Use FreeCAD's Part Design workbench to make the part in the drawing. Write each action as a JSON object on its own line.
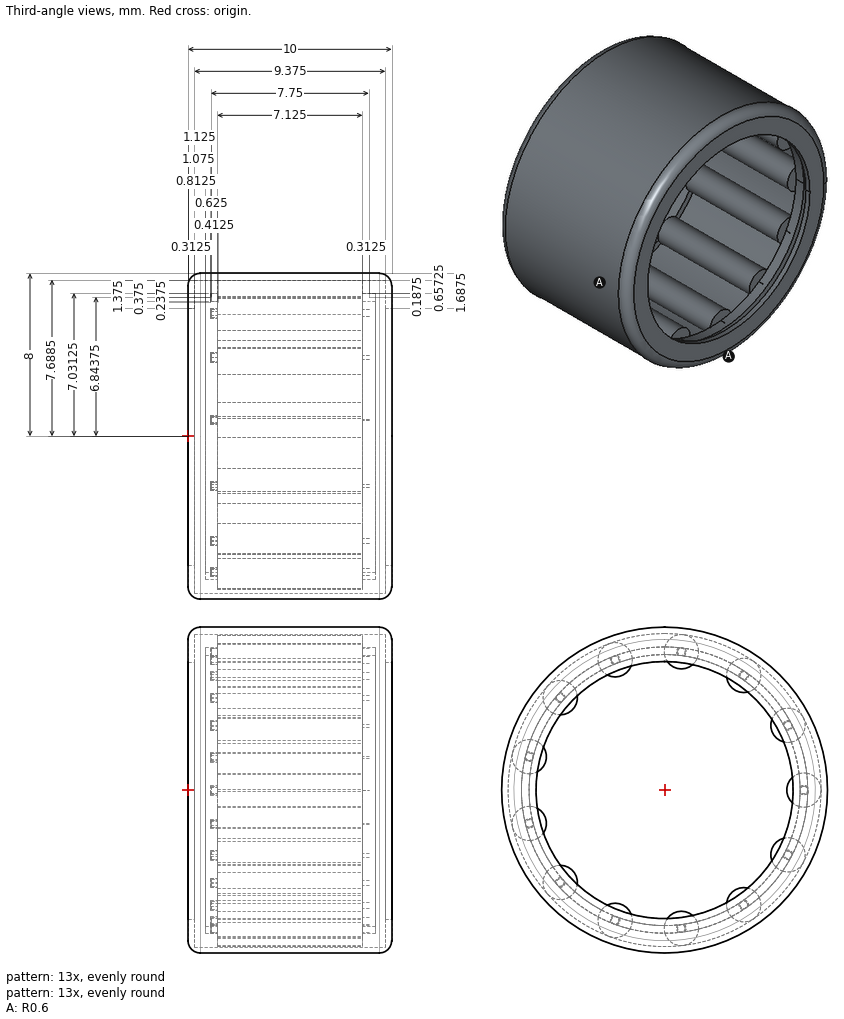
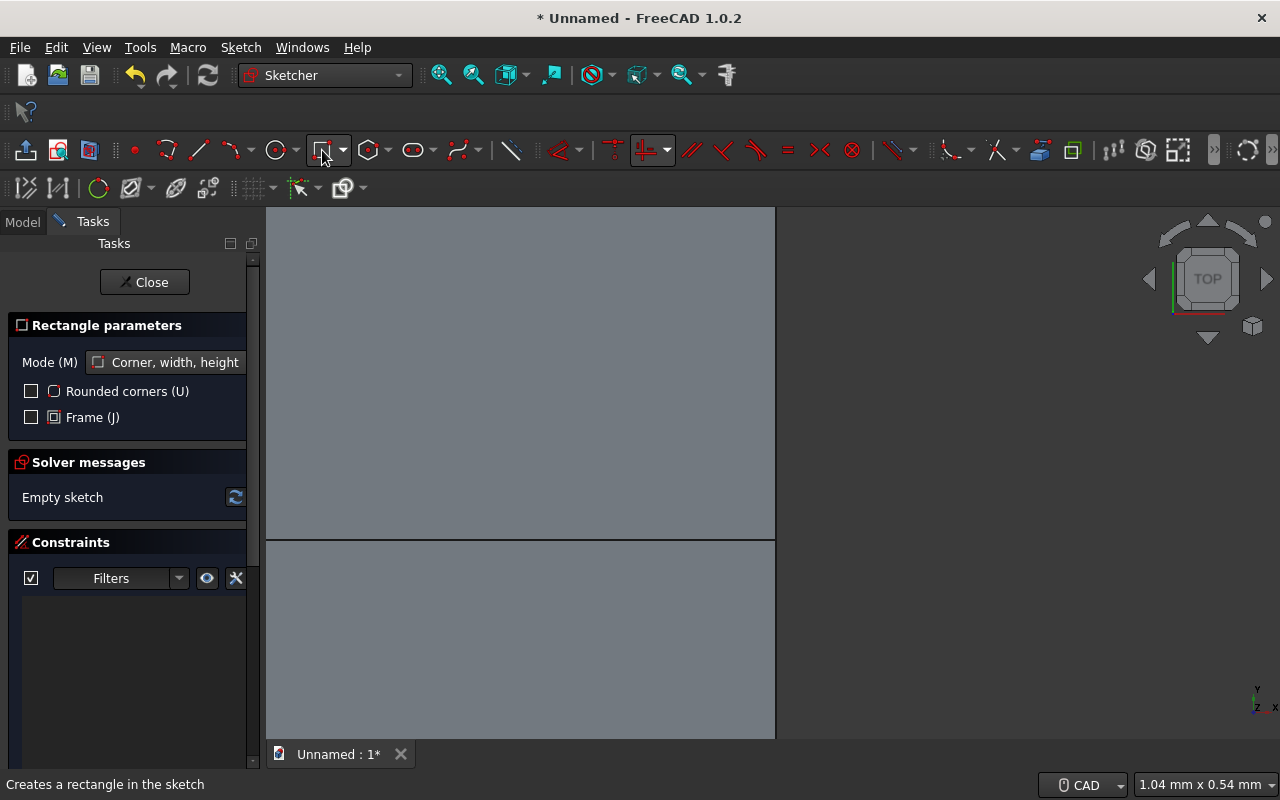
{"action": "left_click", "coordinate": [421, 356]}
{"action": "left_click", "coordinate": [825, 589]}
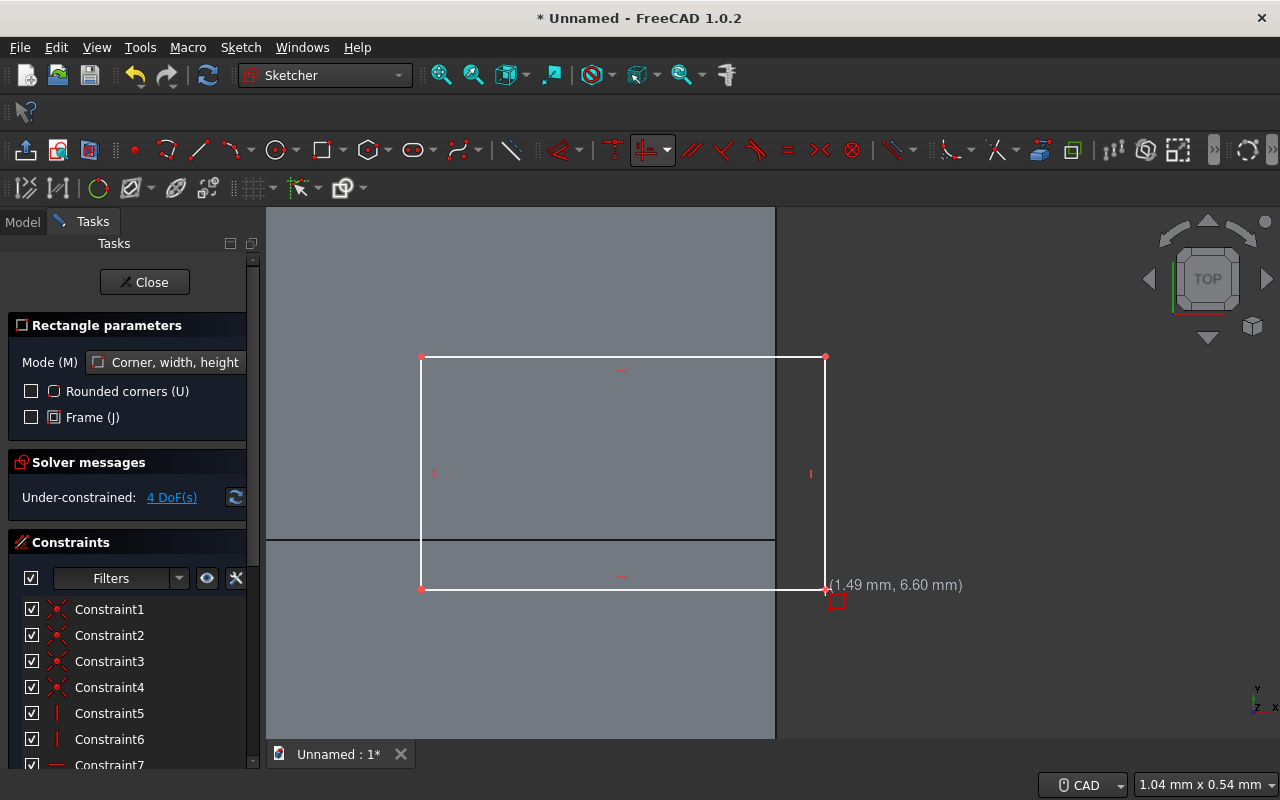
{"action": "left_click", "coordinate": [200, 150]}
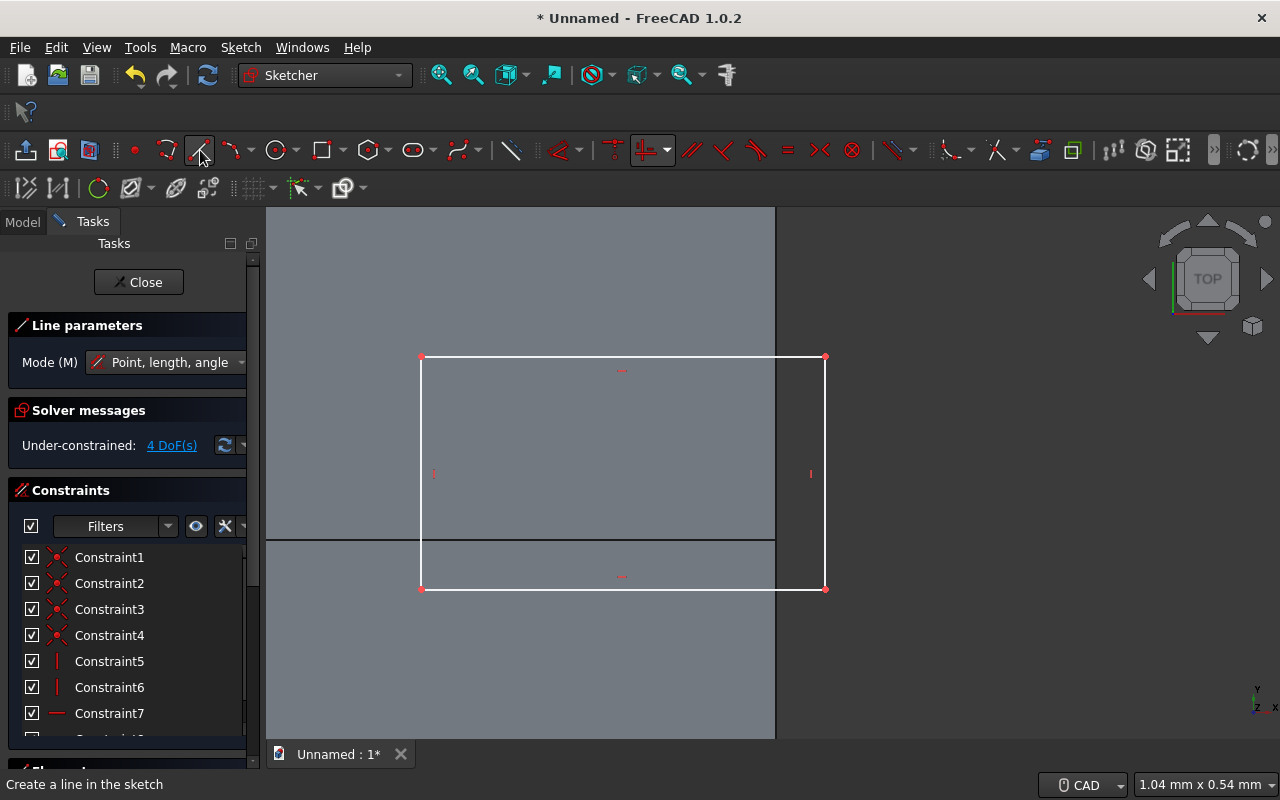
{"action": "left_click", "coordinate": [866, 356]}
{"action": "left_click", "coordinate": [987, 356]}
{"action": "key", "text": "Escape"}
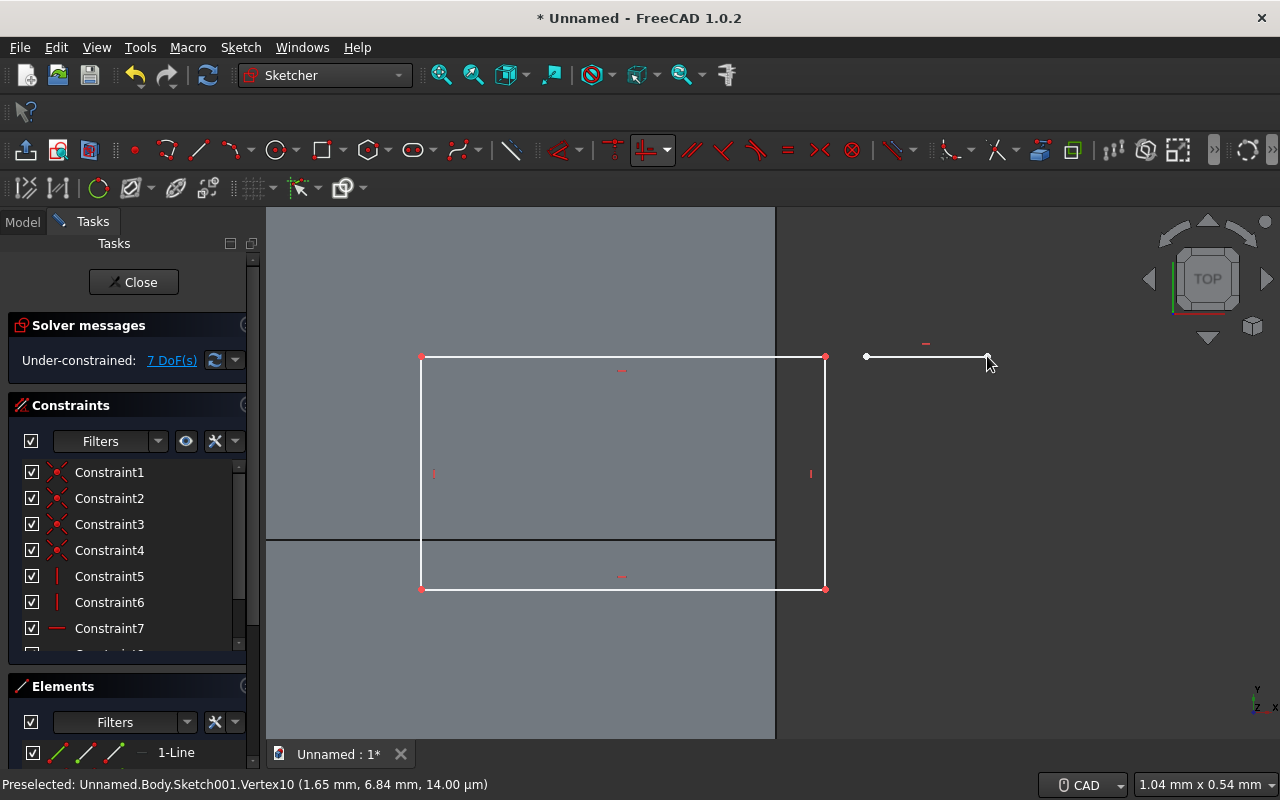
{"action": "left_click", "coordinate": [902, 357]}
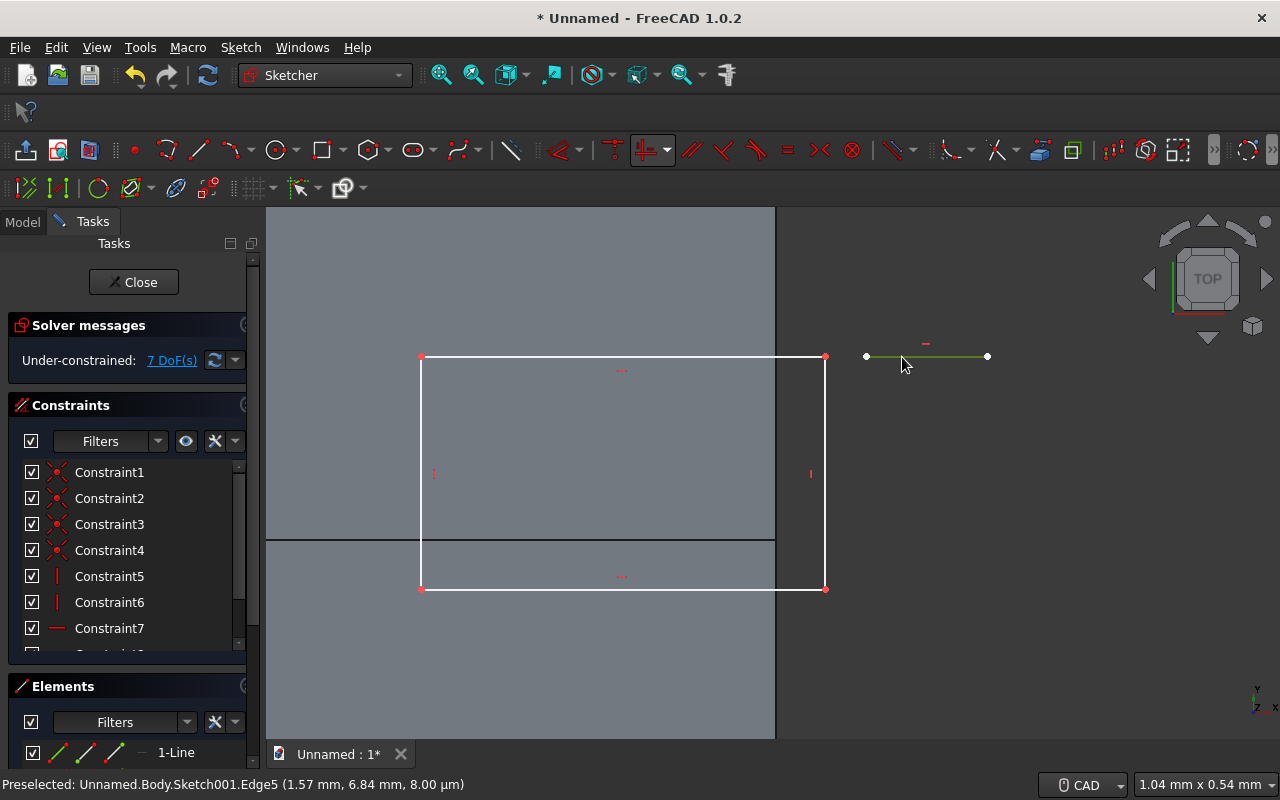
{"action": "left_click", "coordinate": [512, 150]}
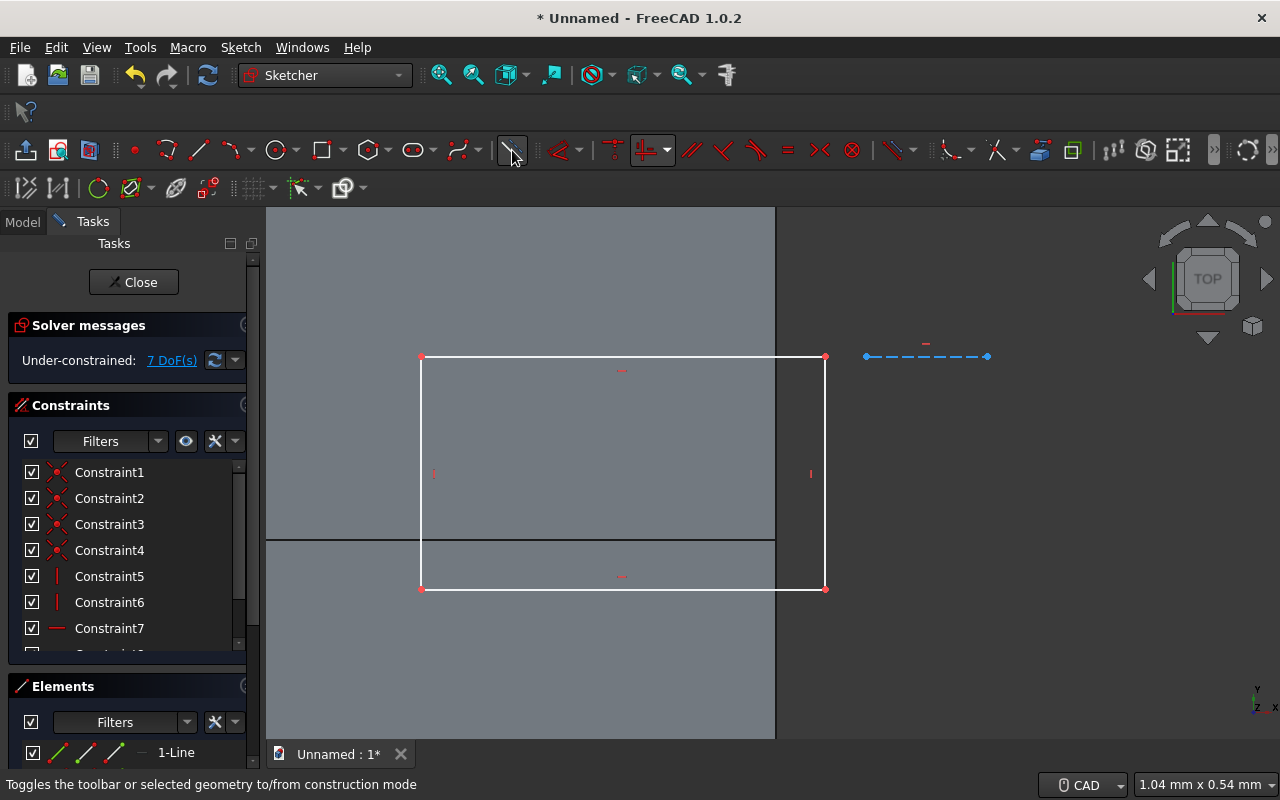
{"action": "left_click", "coordinate": [558, 150]}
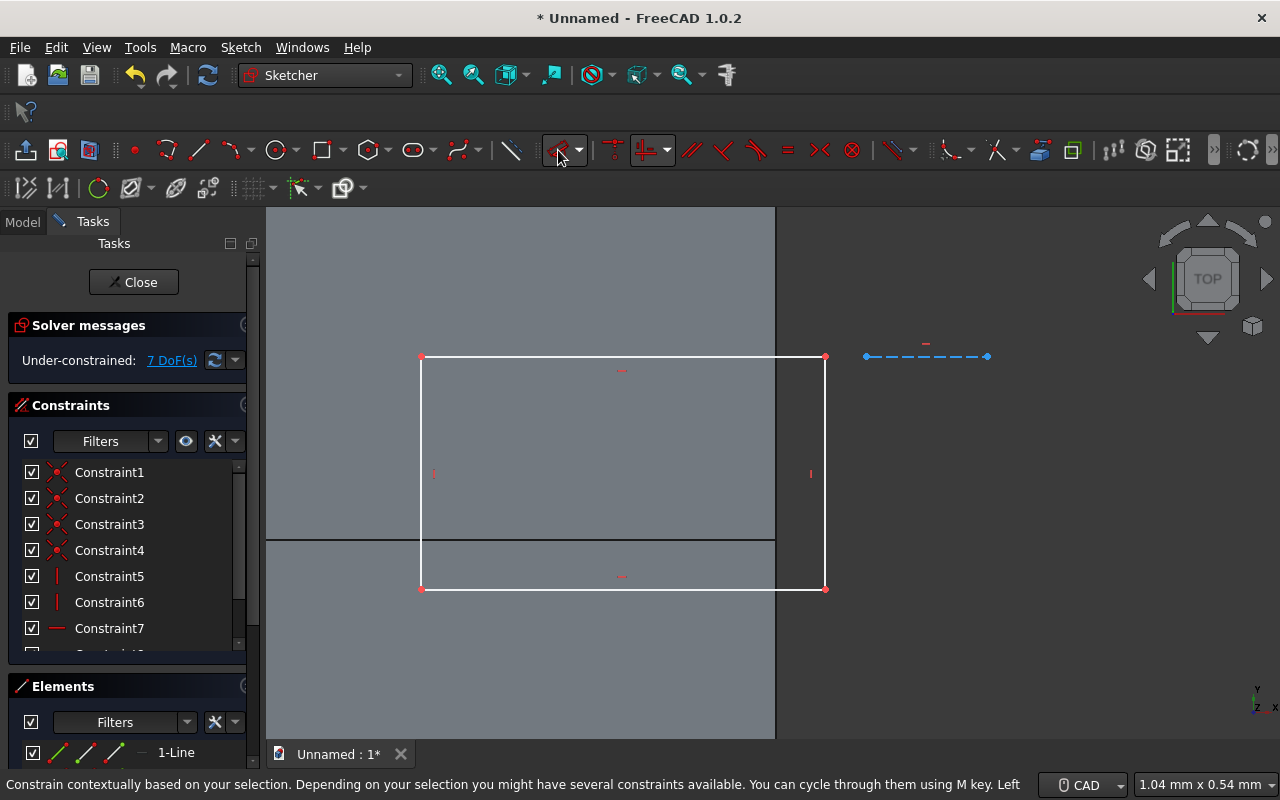
{"action": "left_click", "coordinate": [421, 427]}
{"action": "left_click", "coordinate": [387, 473]}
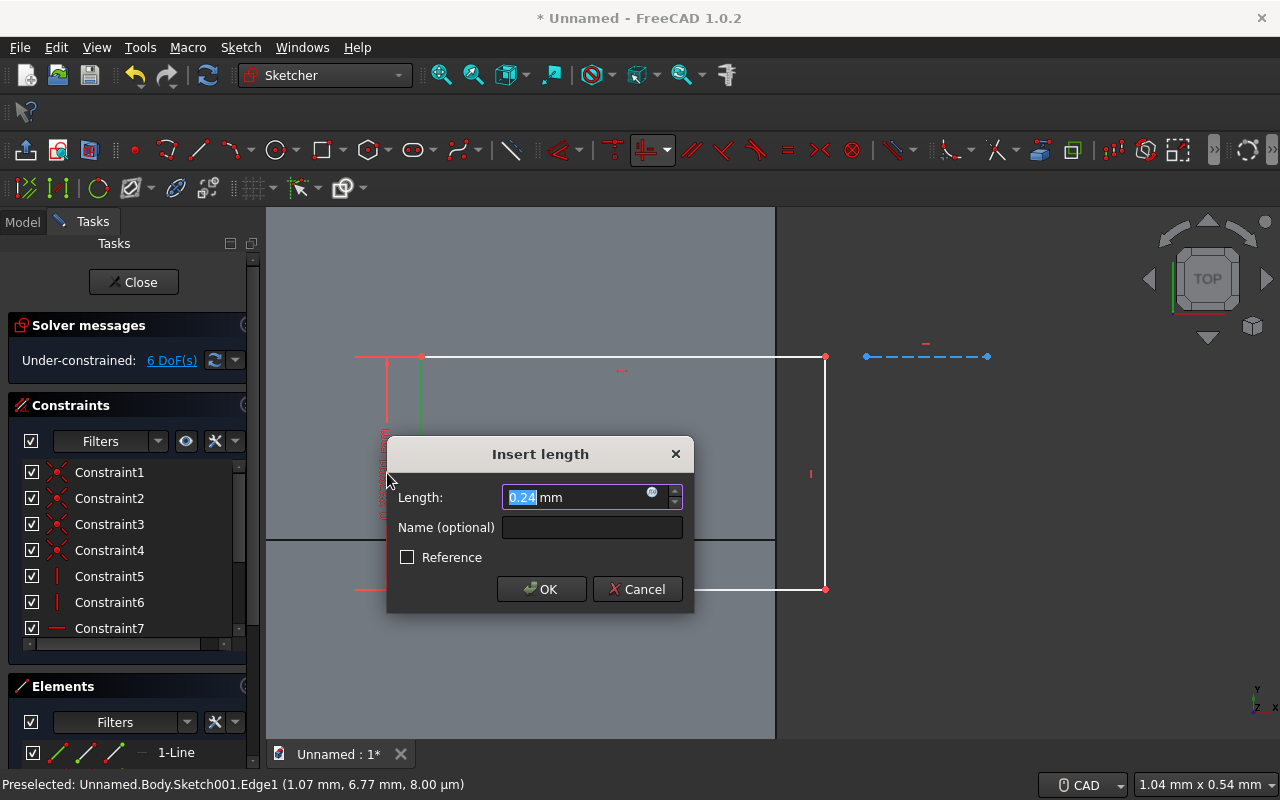
{"action": "type", "text": "0.2375"}
{"action": "key", "text": "Return"}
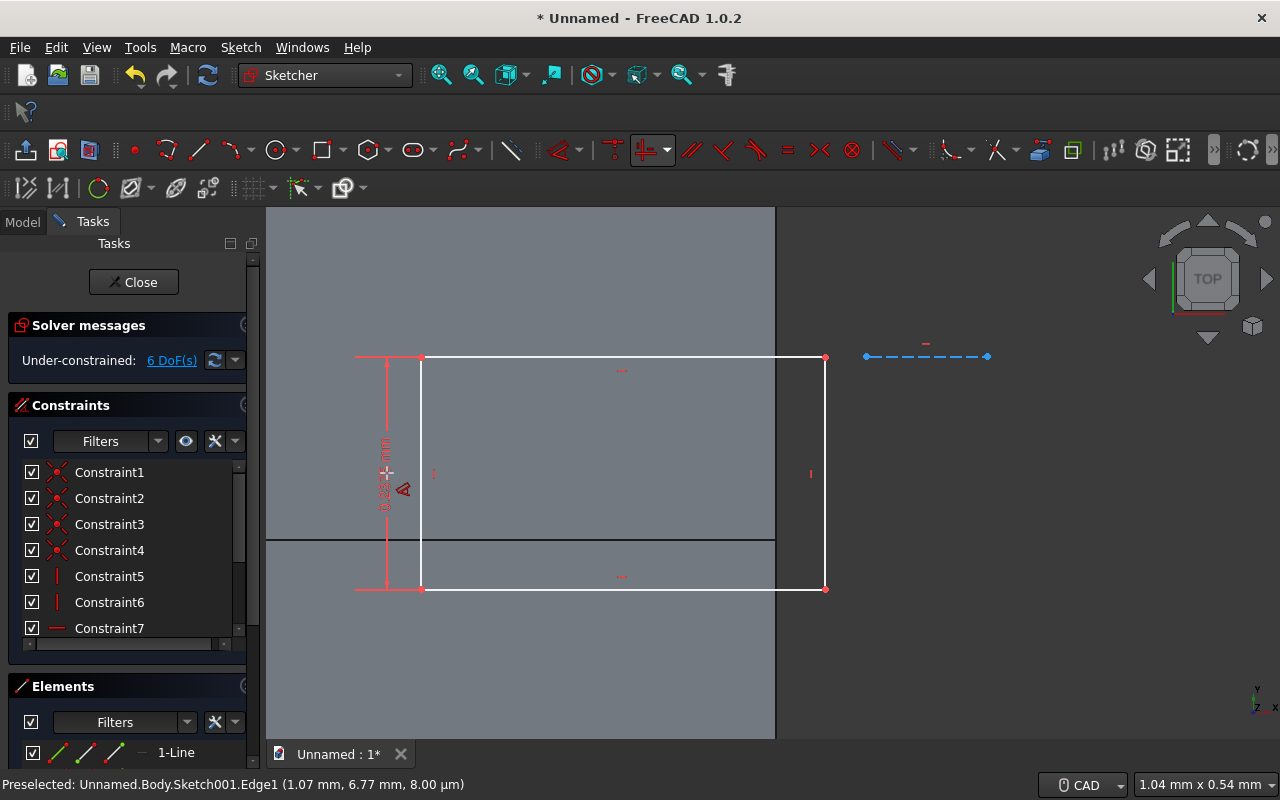
{"action": "left_click", "coordinate": [542, 590]}
{"action": "left_click", "coordinate": [623, 624]}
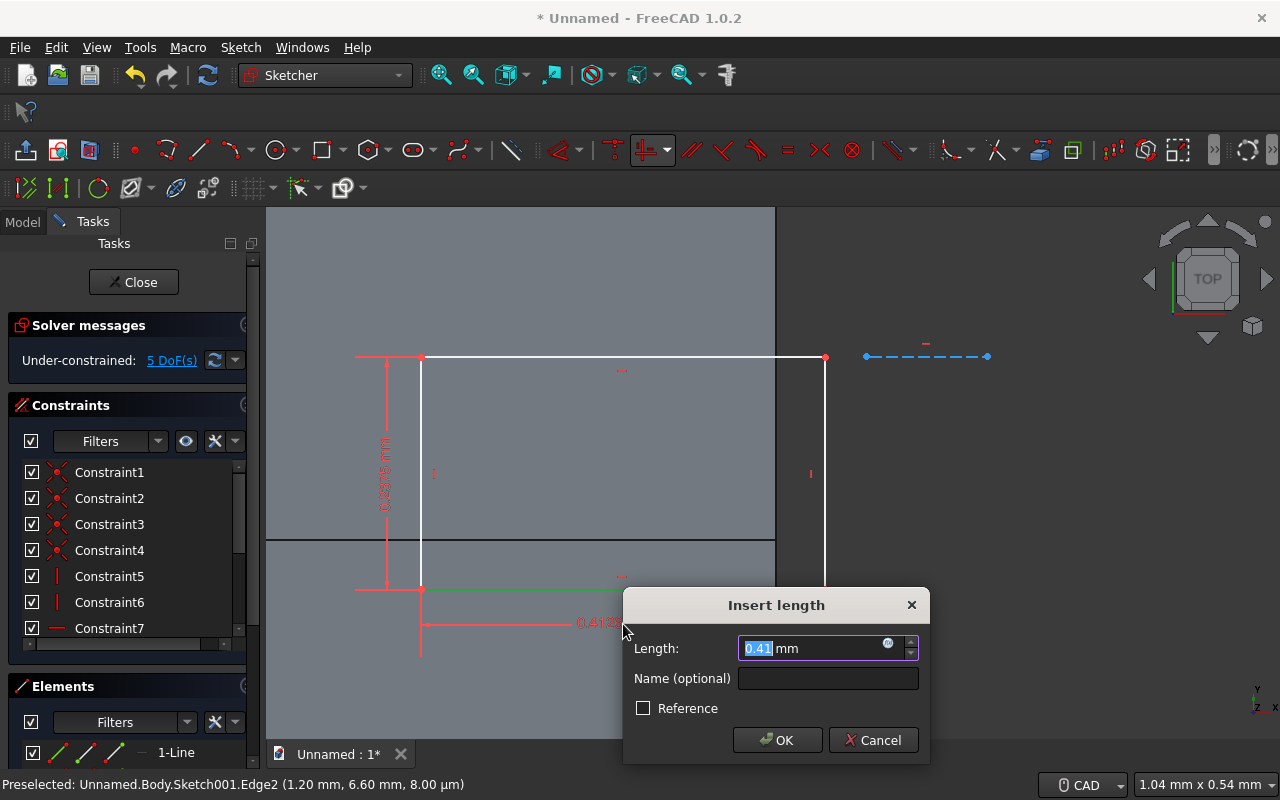
{"action": "type", "text": "0.4125"}
{"action": "key", "text": "Return"}